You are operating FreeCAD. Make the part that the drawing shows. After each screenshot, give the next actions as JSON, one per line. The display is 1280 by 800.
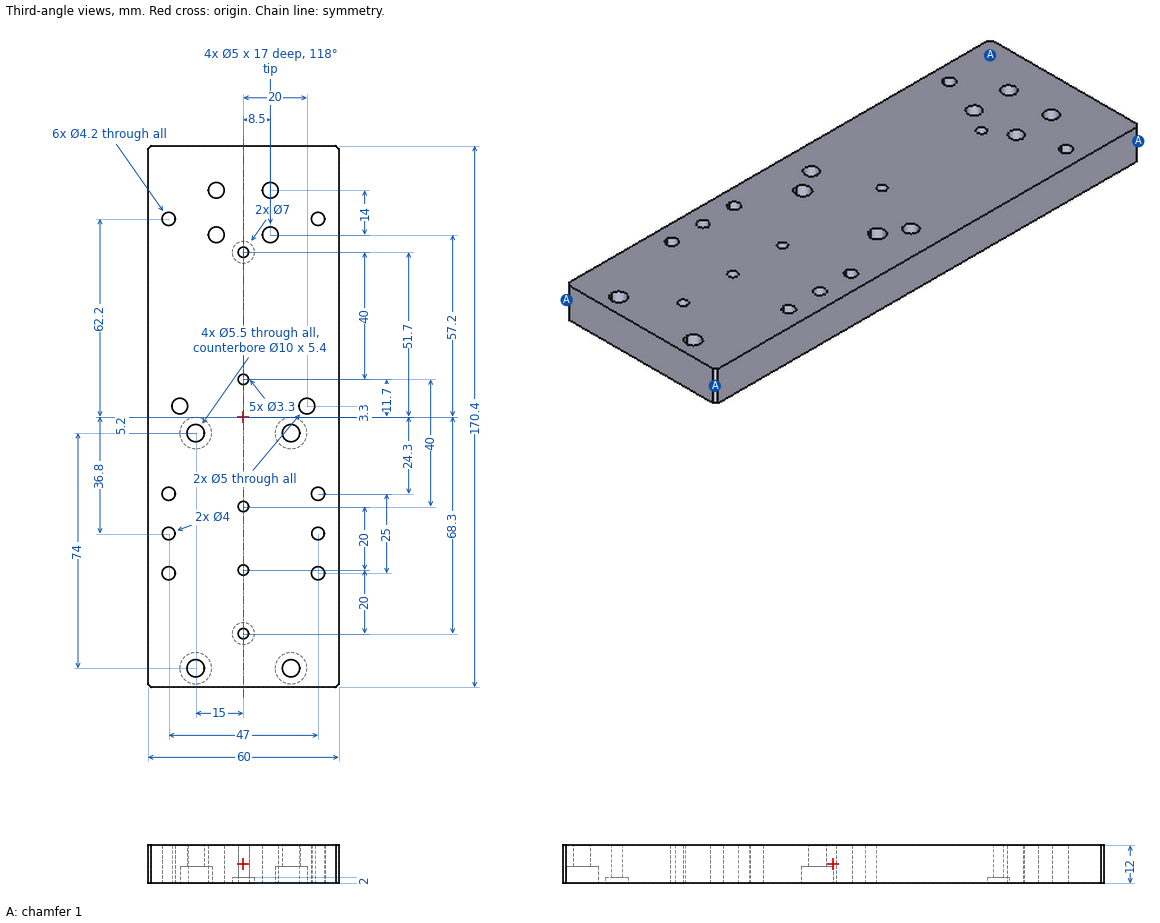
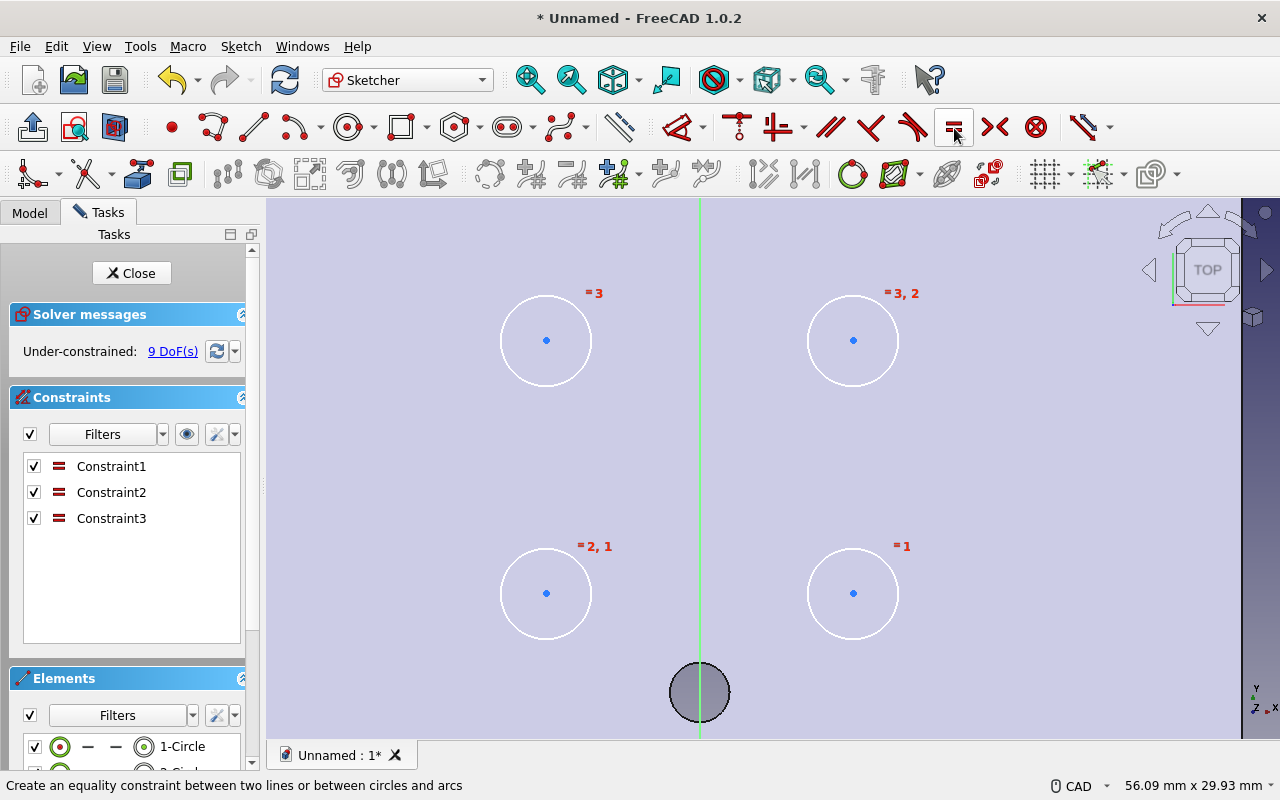
{"action": "left_click", "coordinate": [853, 594]}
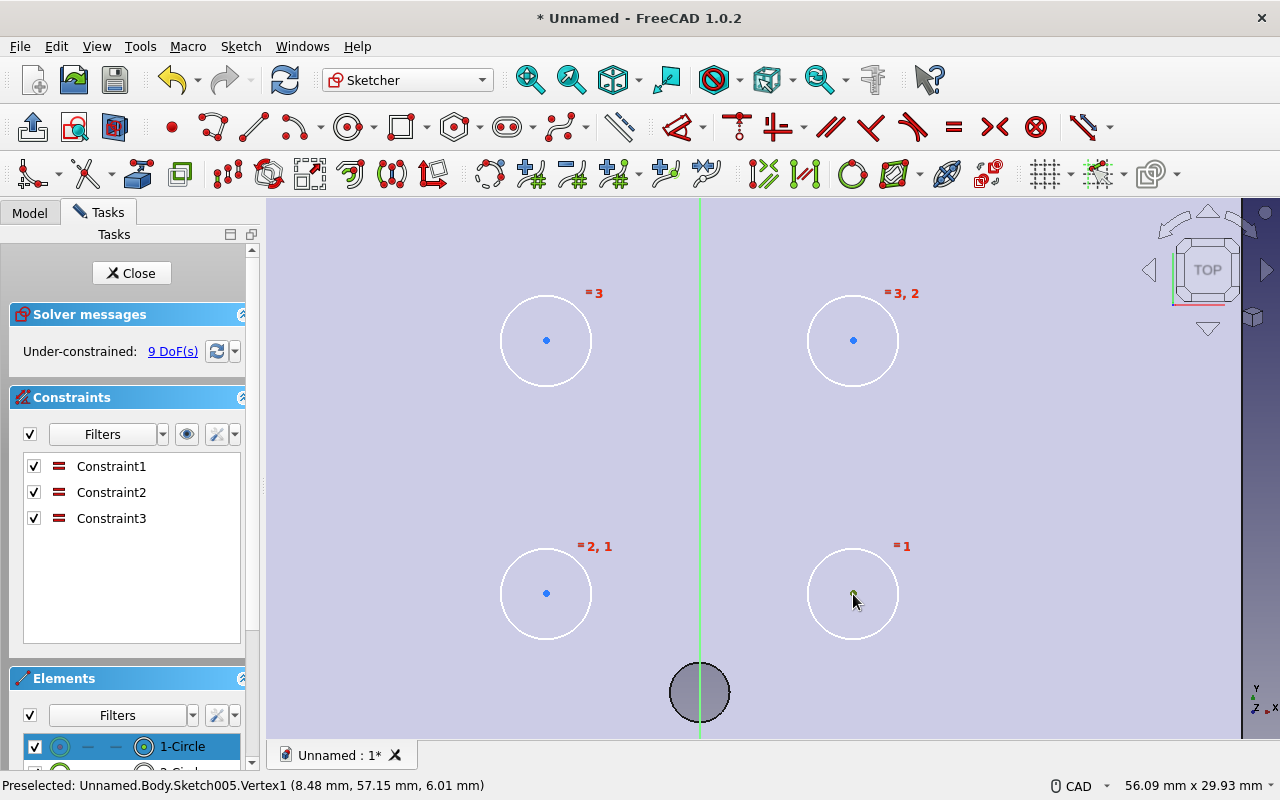
{"action": "left_click", "coordinate": [546, 594]}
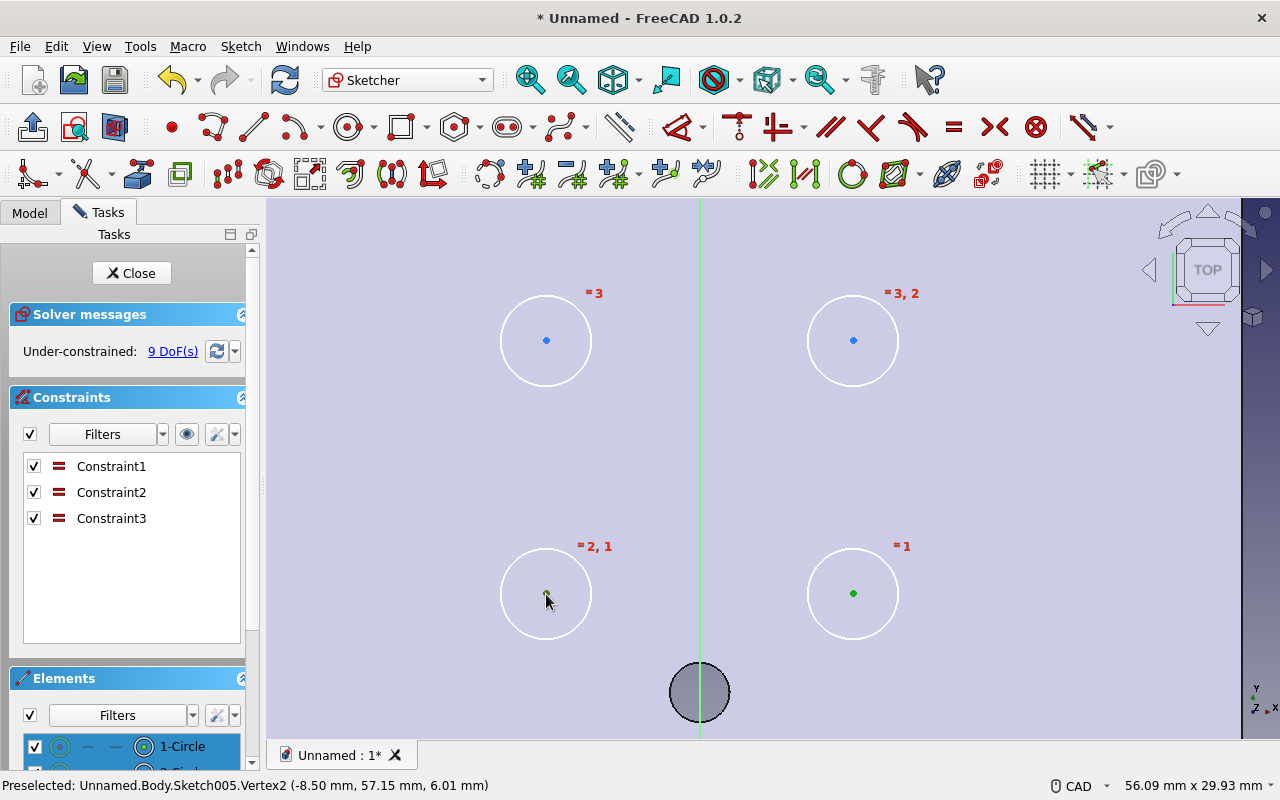
{"action": "left_click", "coordinate": [700, 676]}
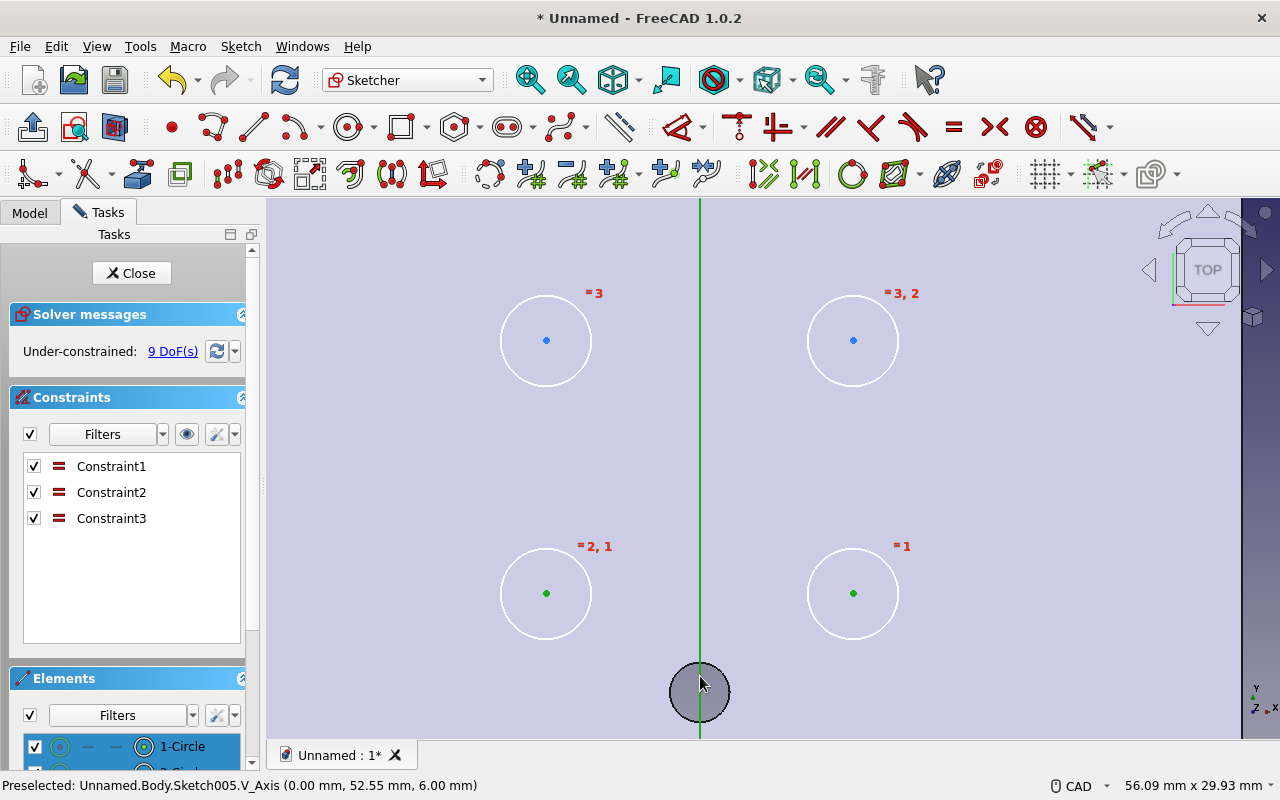
{"action": "left_click", "coordinate": [995, 128]}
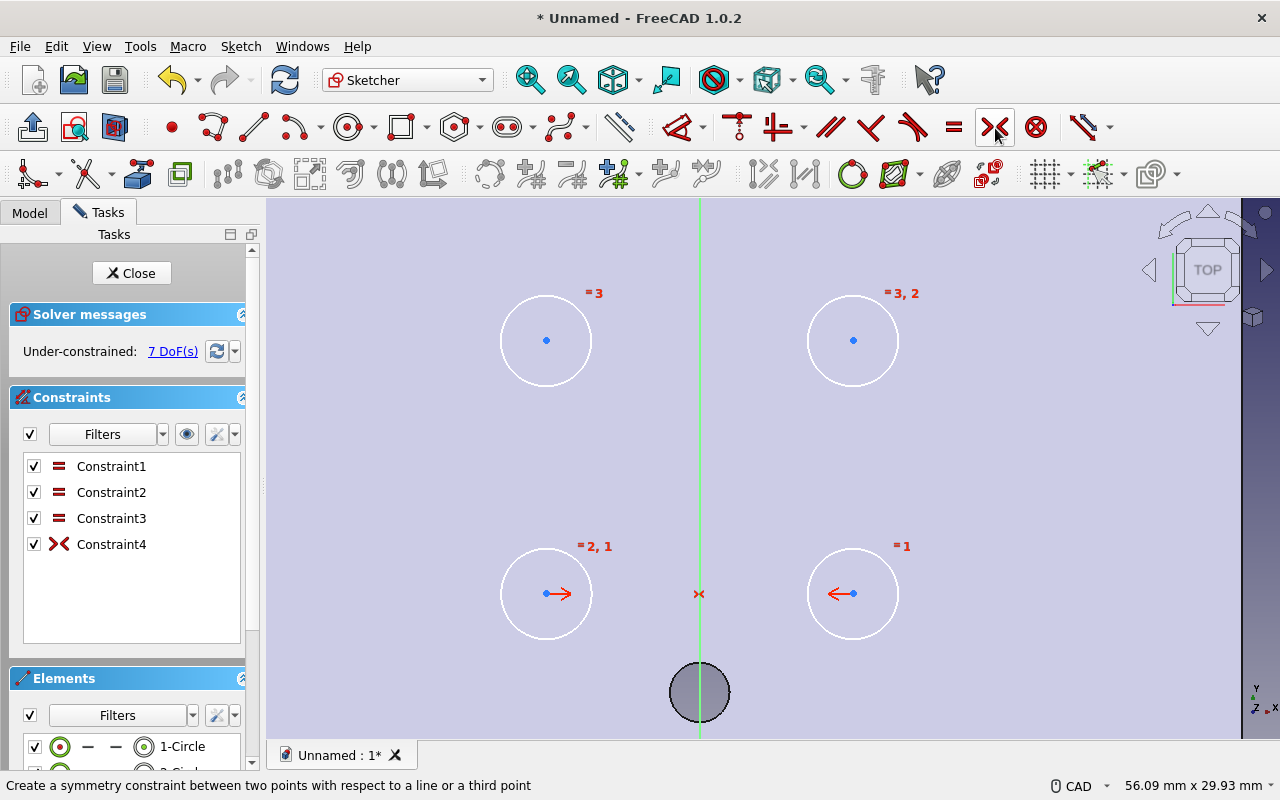
{"action": "left_click", "coordinate": [853, 341]}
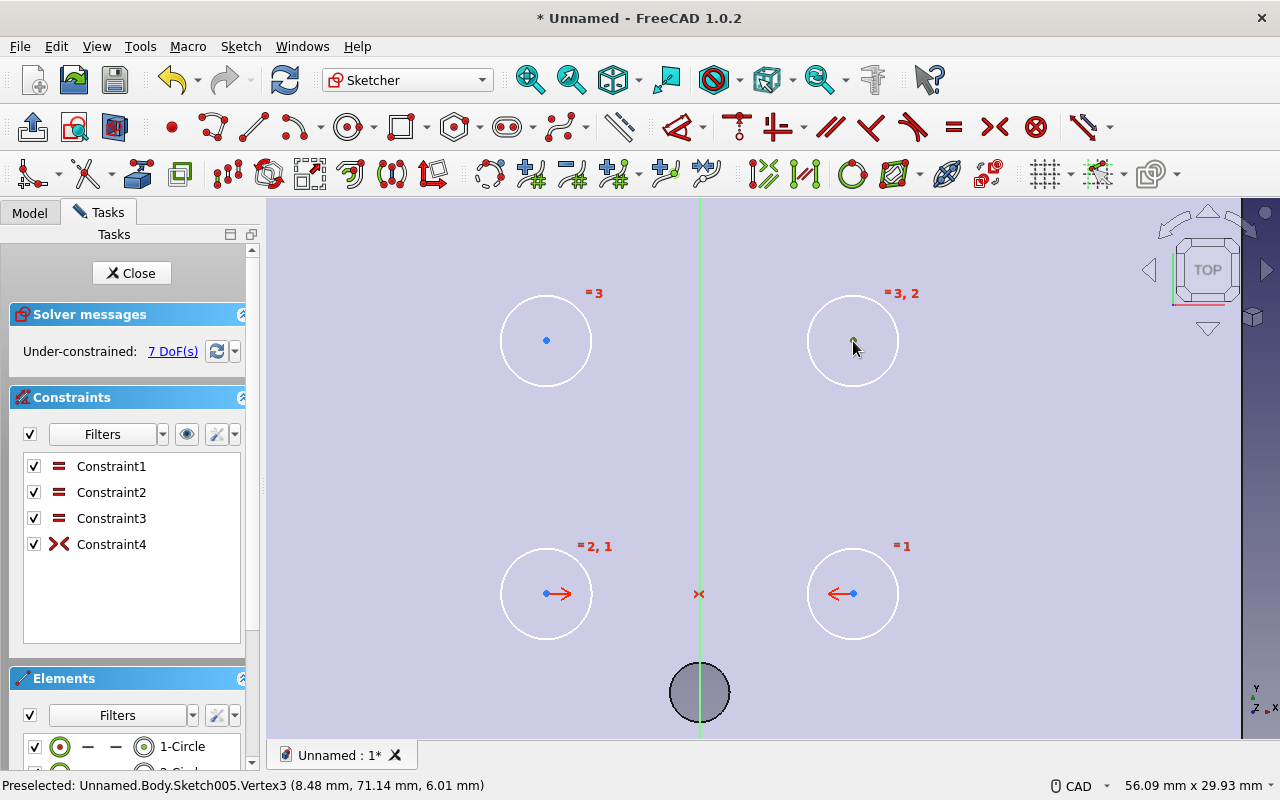
{"action": "left_click", "coordinate": [546, 341]}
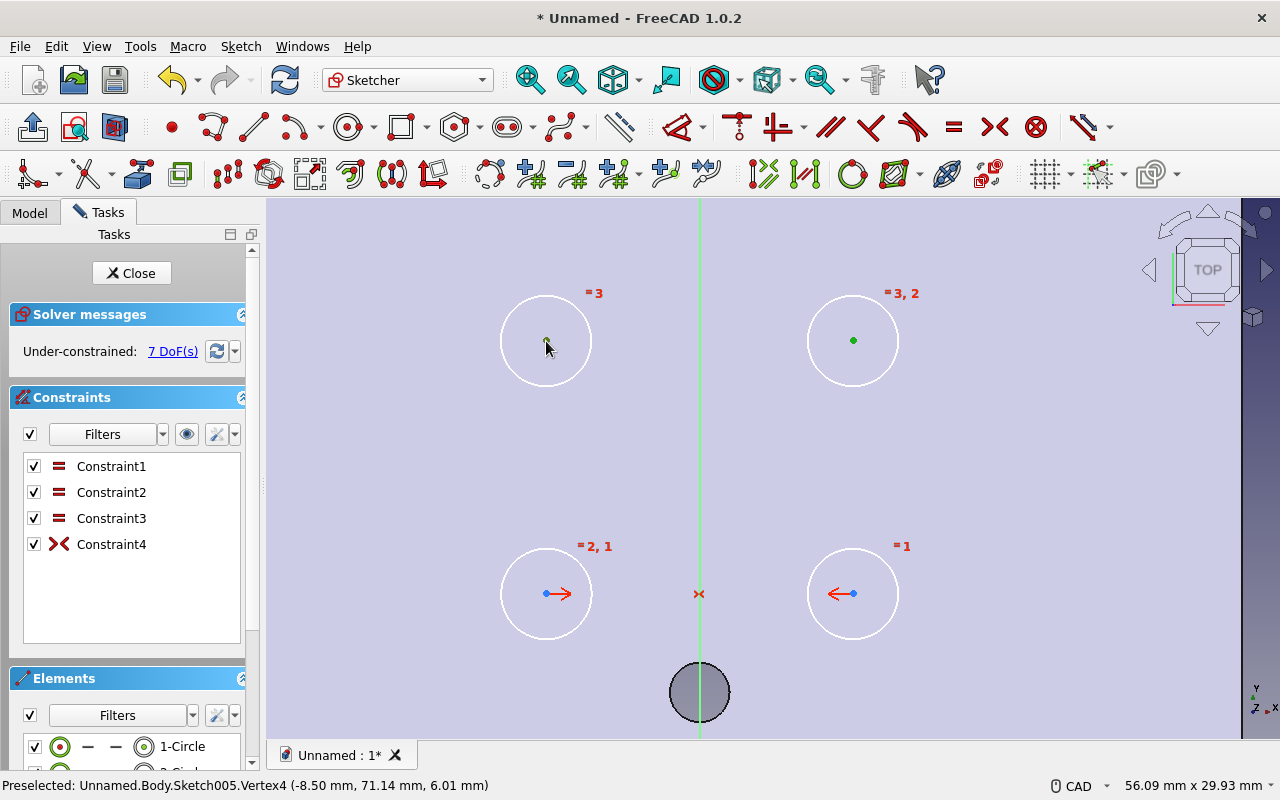
{"action": "left_click", "coordinate": [700, 676]}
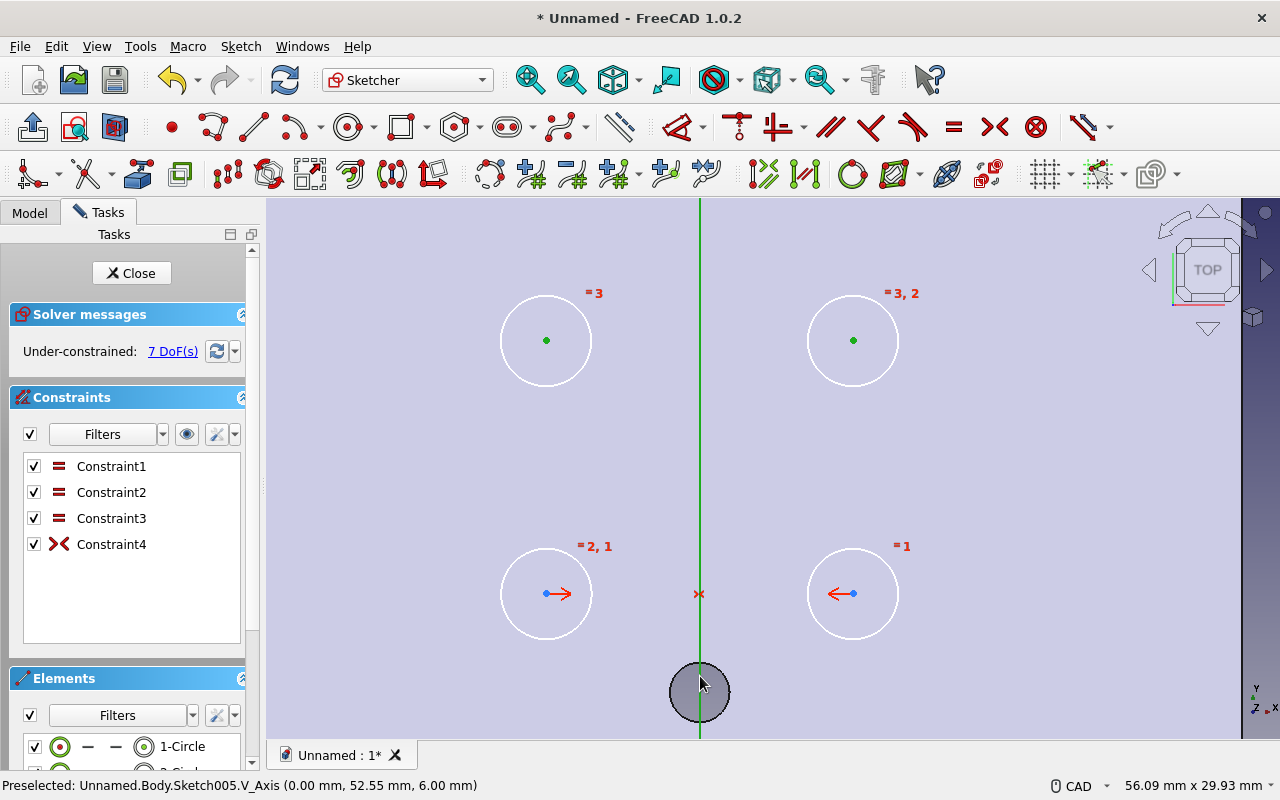
{"action": "left_click", "coordinate": [995, 128]}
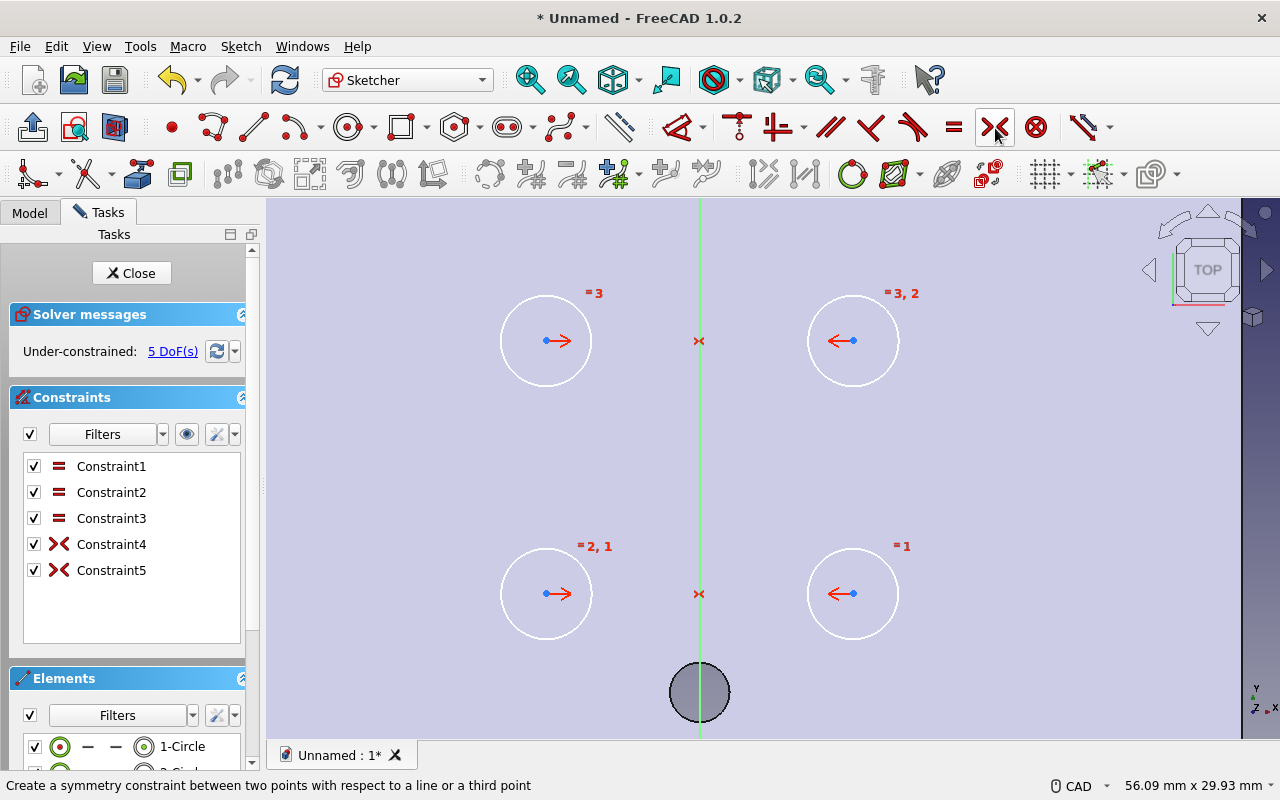
{"action": "key", "text": "d"}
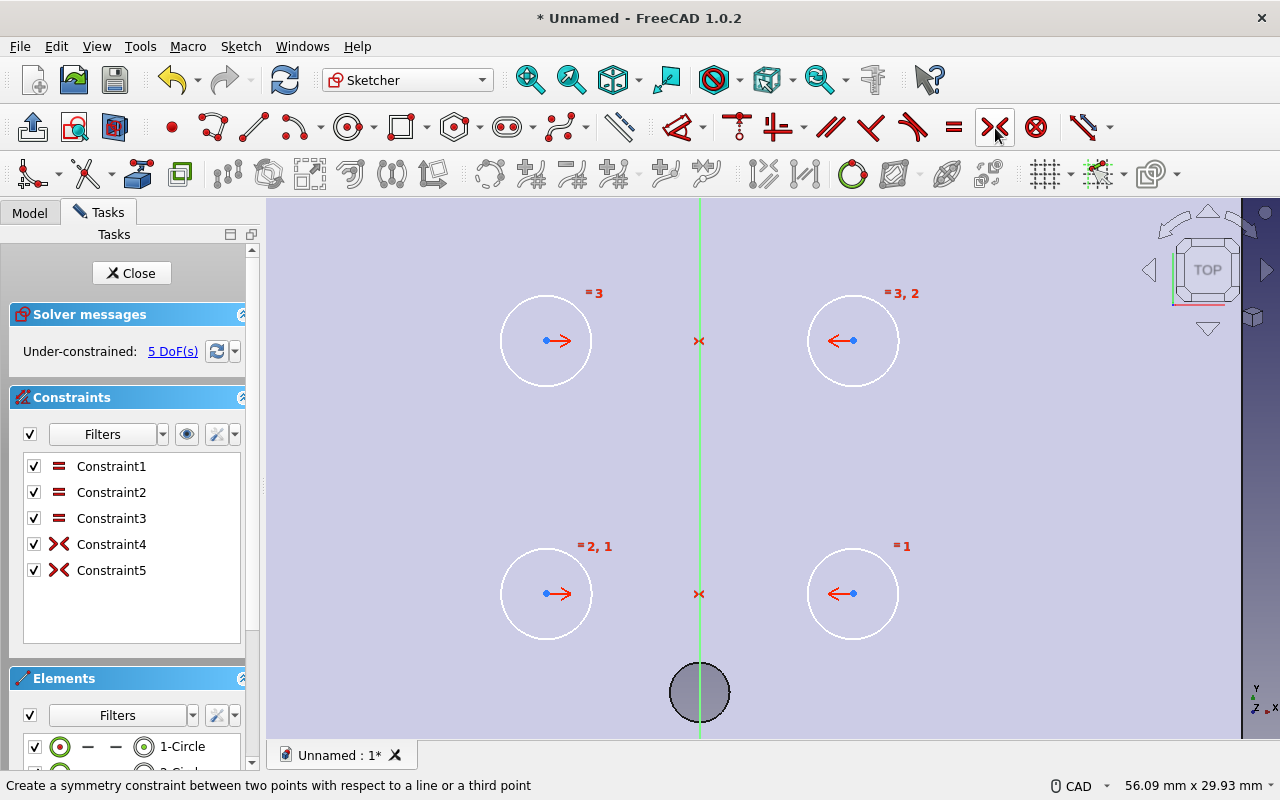
{"action": "left_click", "coordinate": [885, 562]}
{"action": "left_click", "coordinate": [908, 539]}